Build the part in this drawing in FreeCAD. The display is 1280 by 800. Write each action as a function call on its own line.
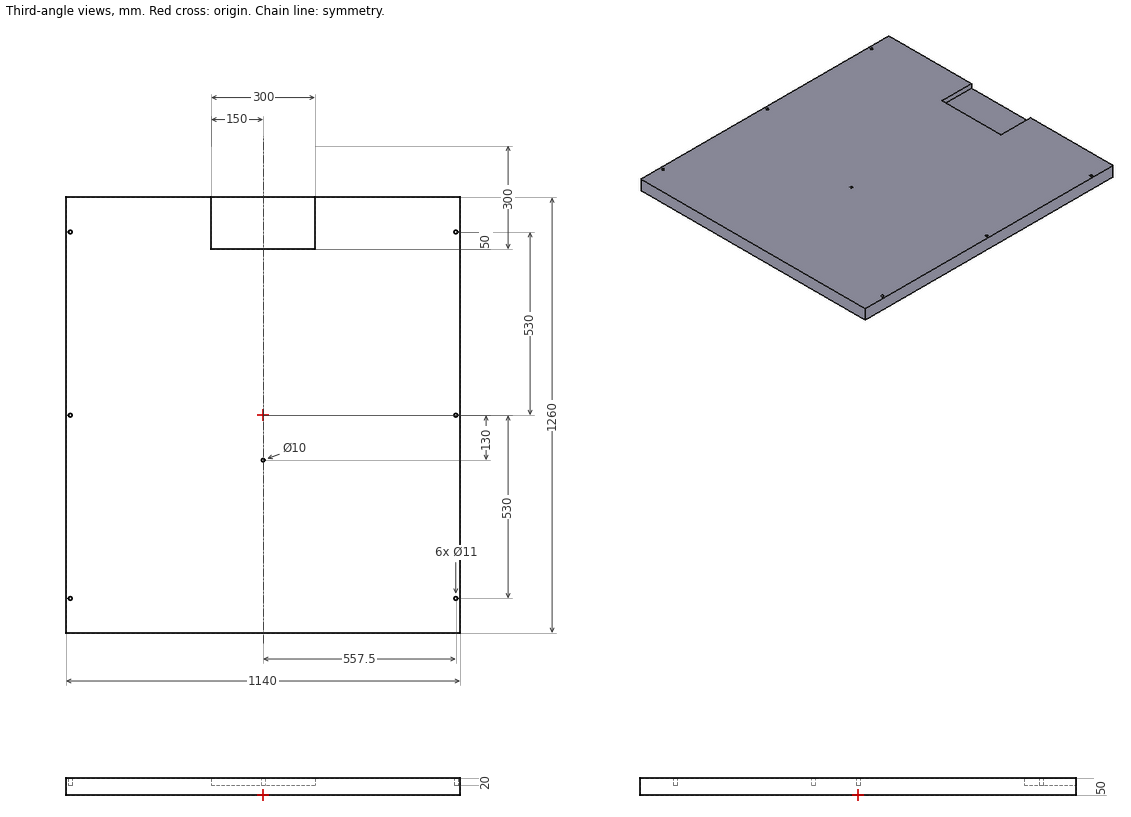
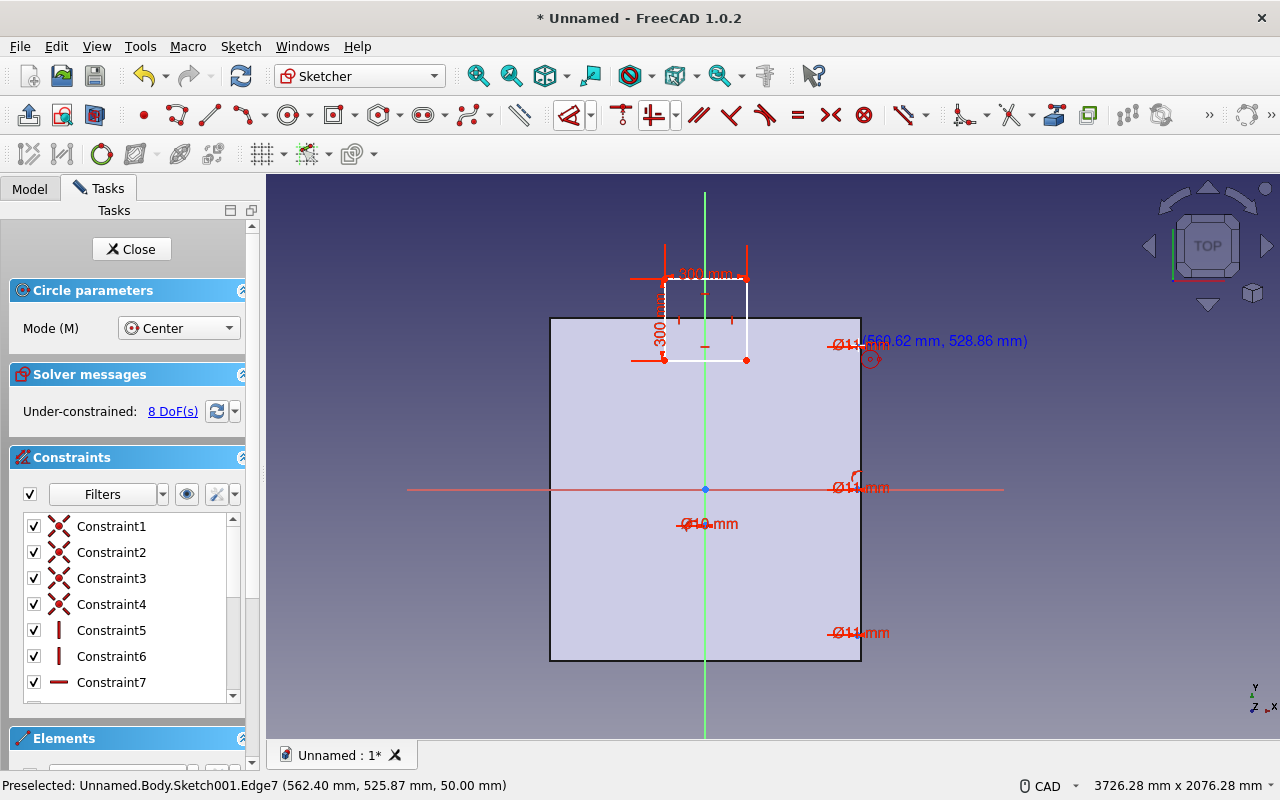
scroll(554, 346, up, 14)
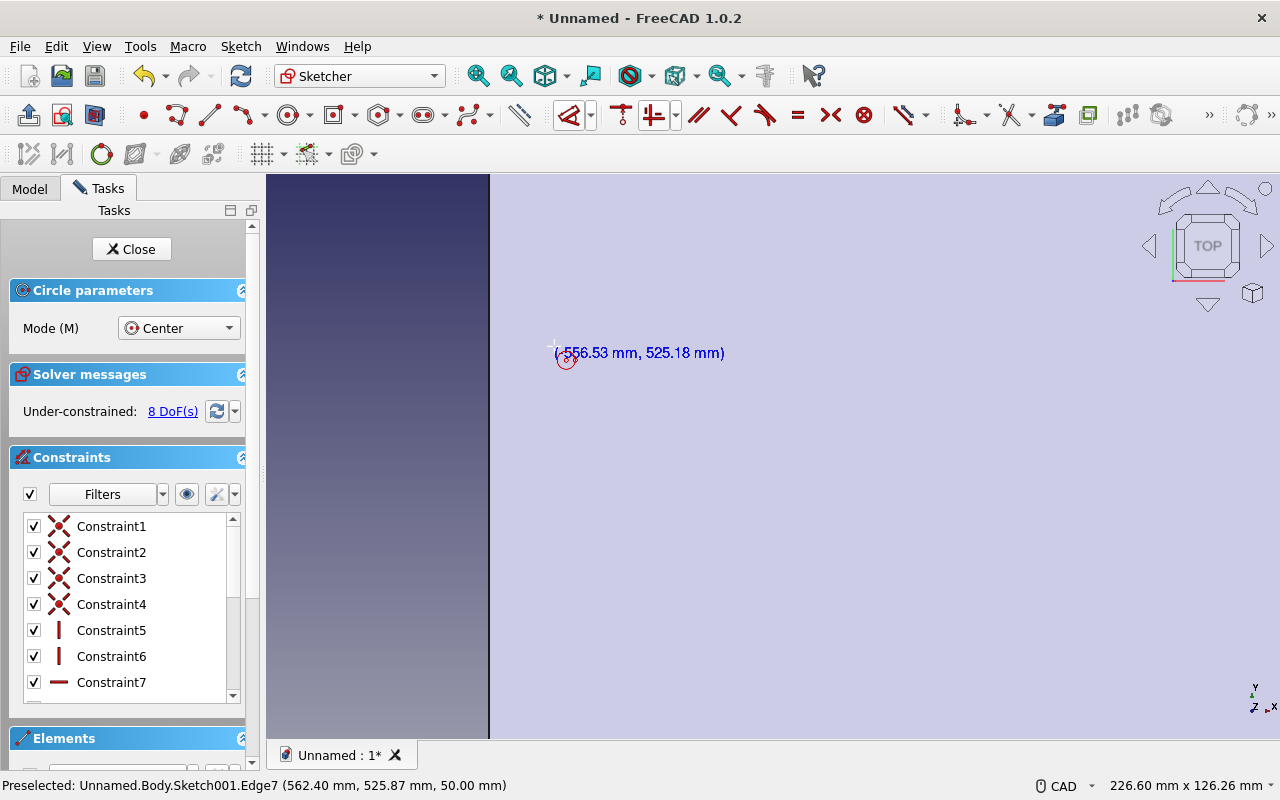
scroll(553, 346, down, 14)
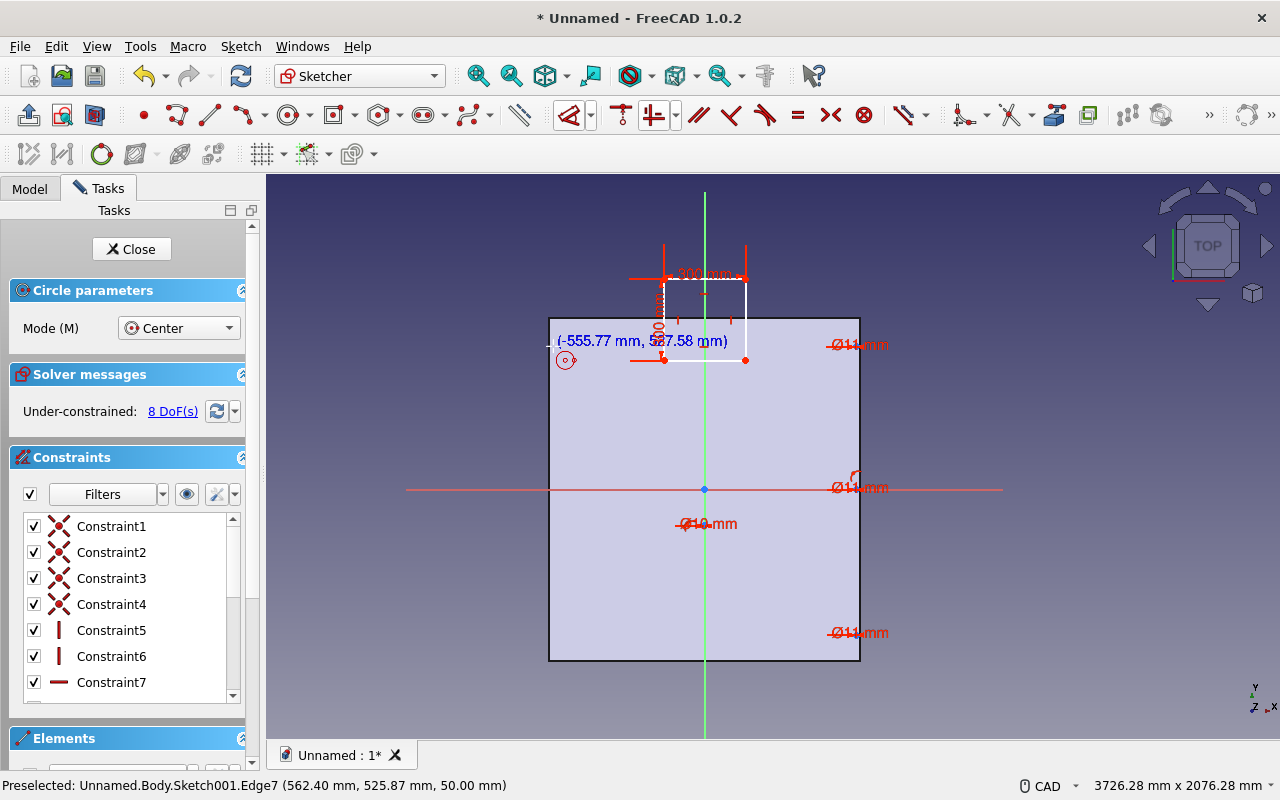
click(553, 346)
move(554, 345)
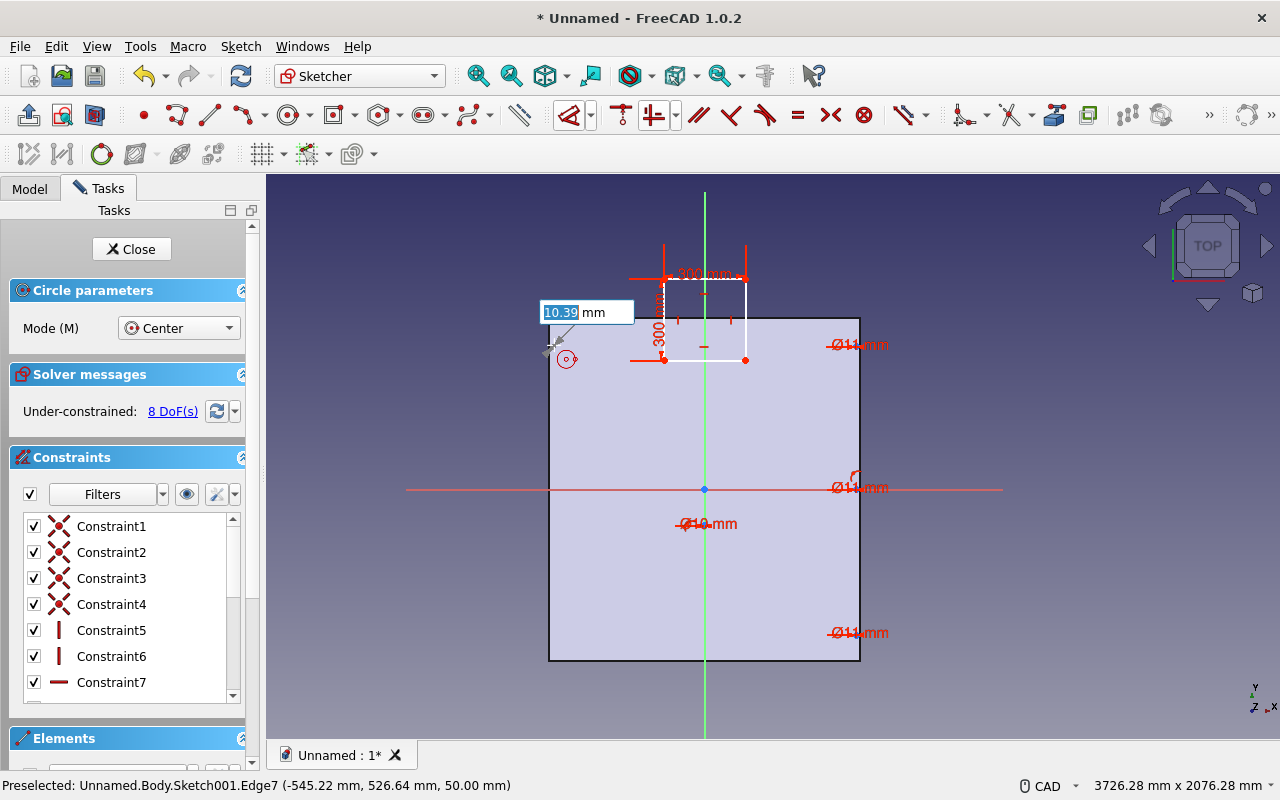
text(11)
key(Return)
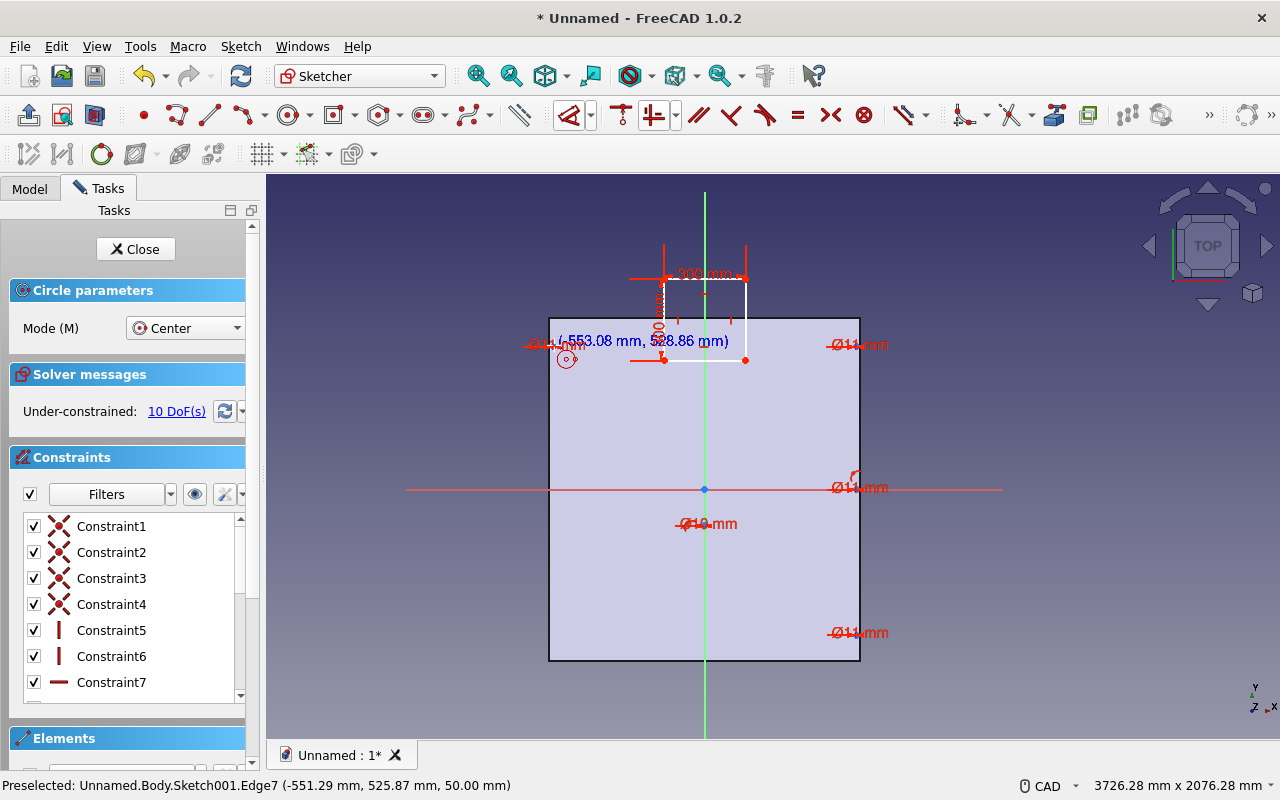
scroll(553, 490, up, 14)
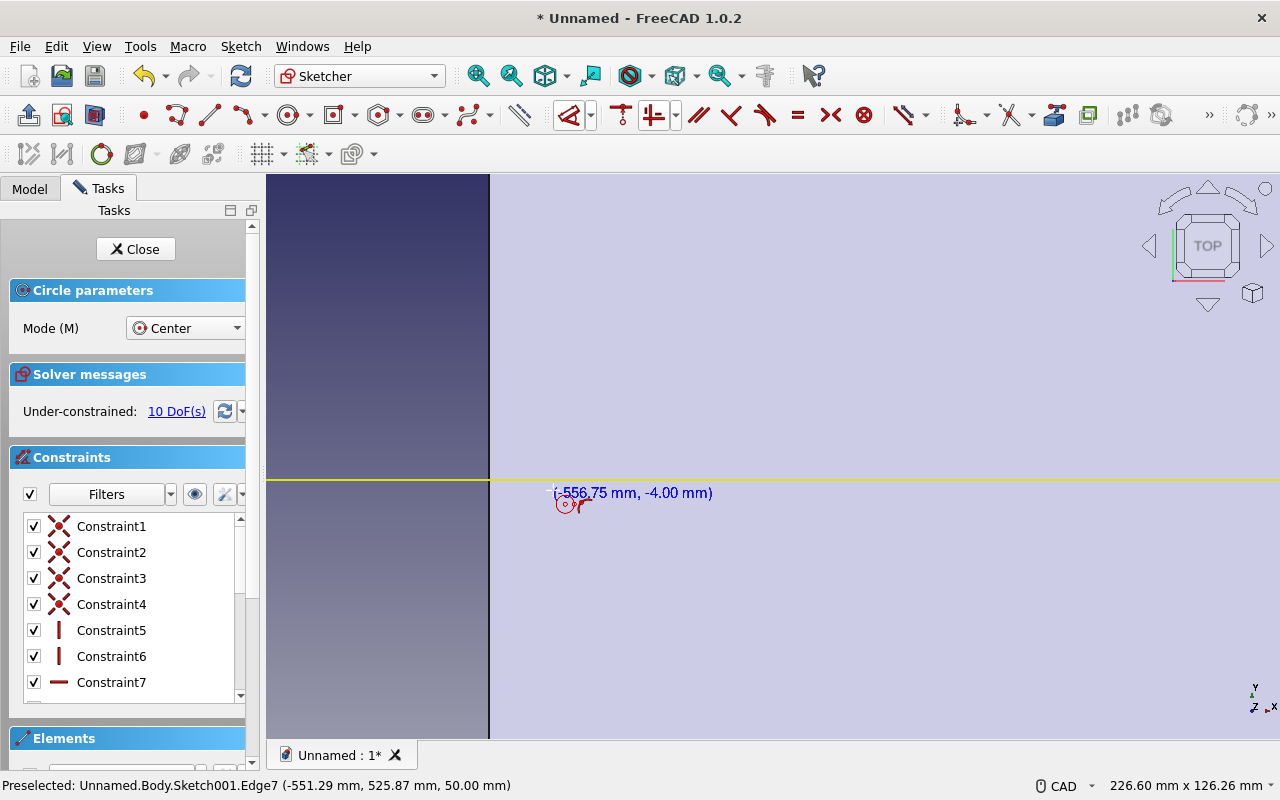
scroll(553, 490, down, 14)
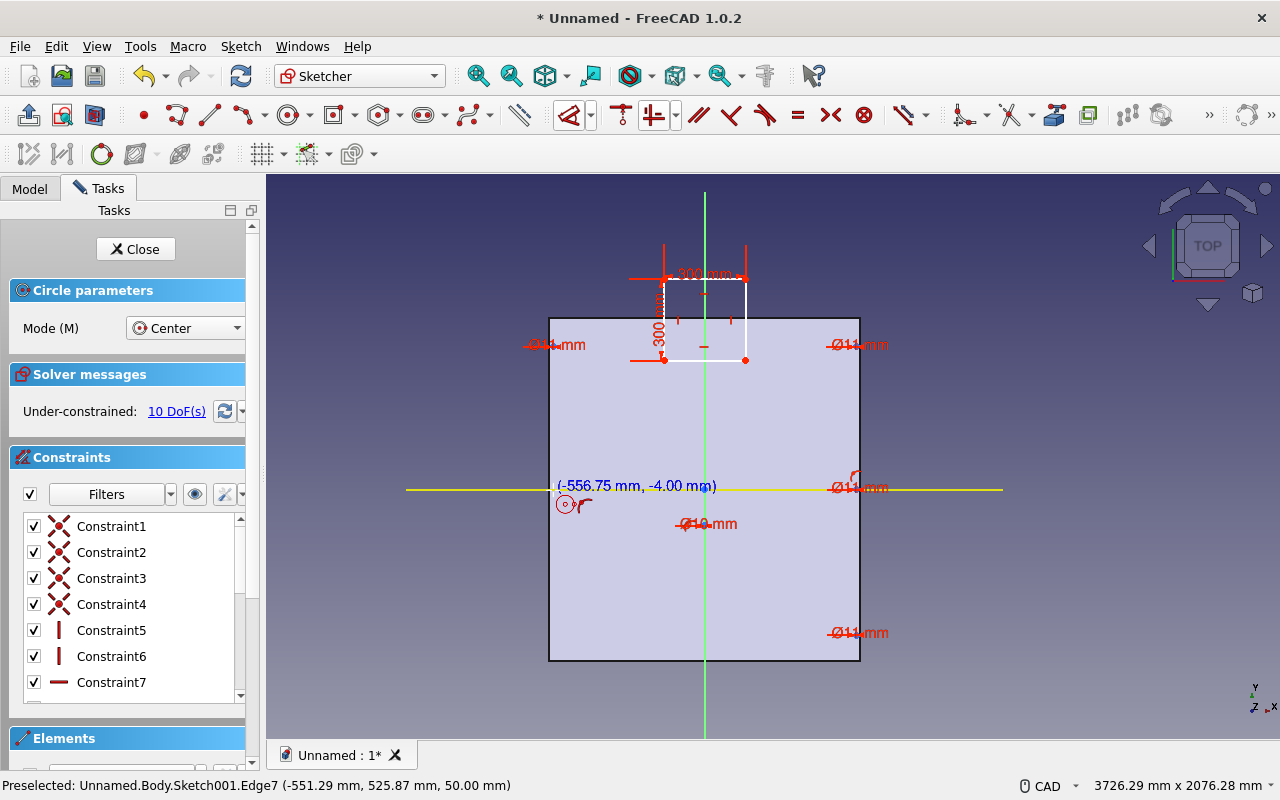
click(553, 490)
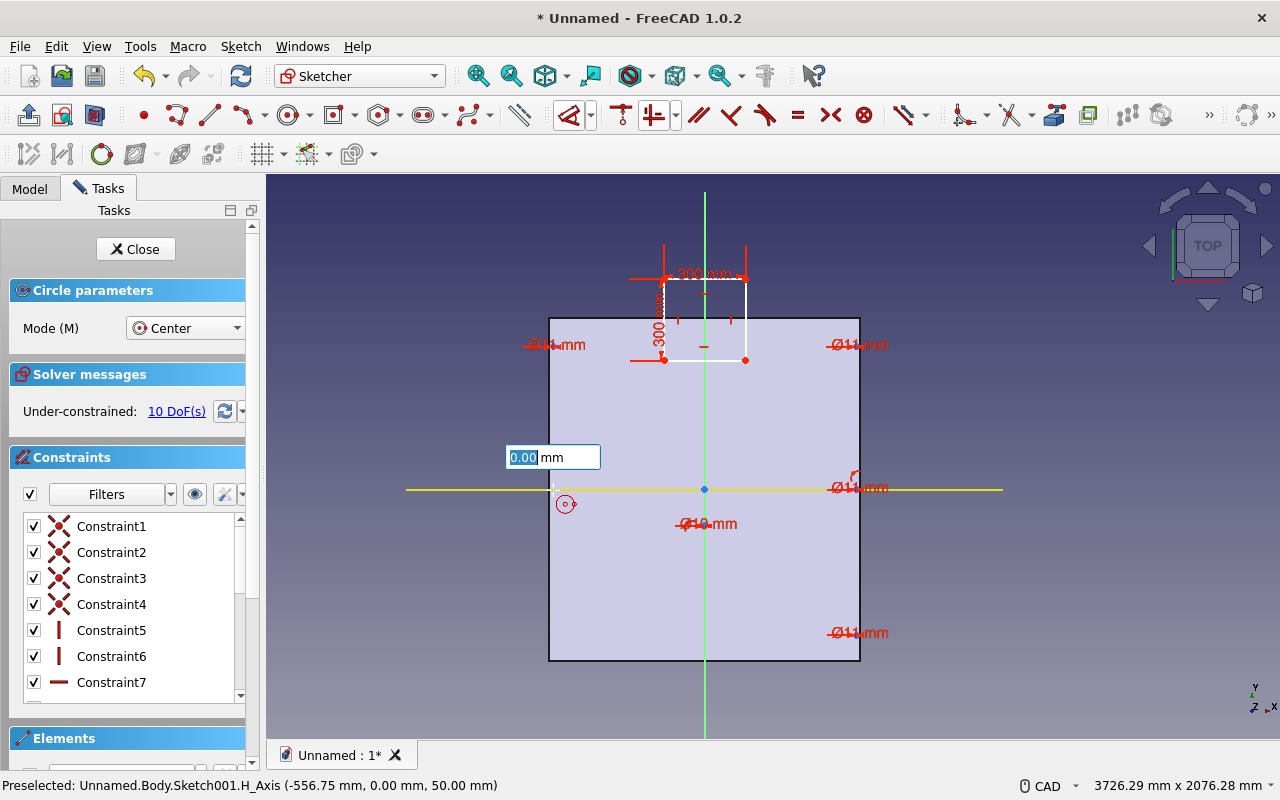
scroll(553, 489, up, 13)
move(554, 475)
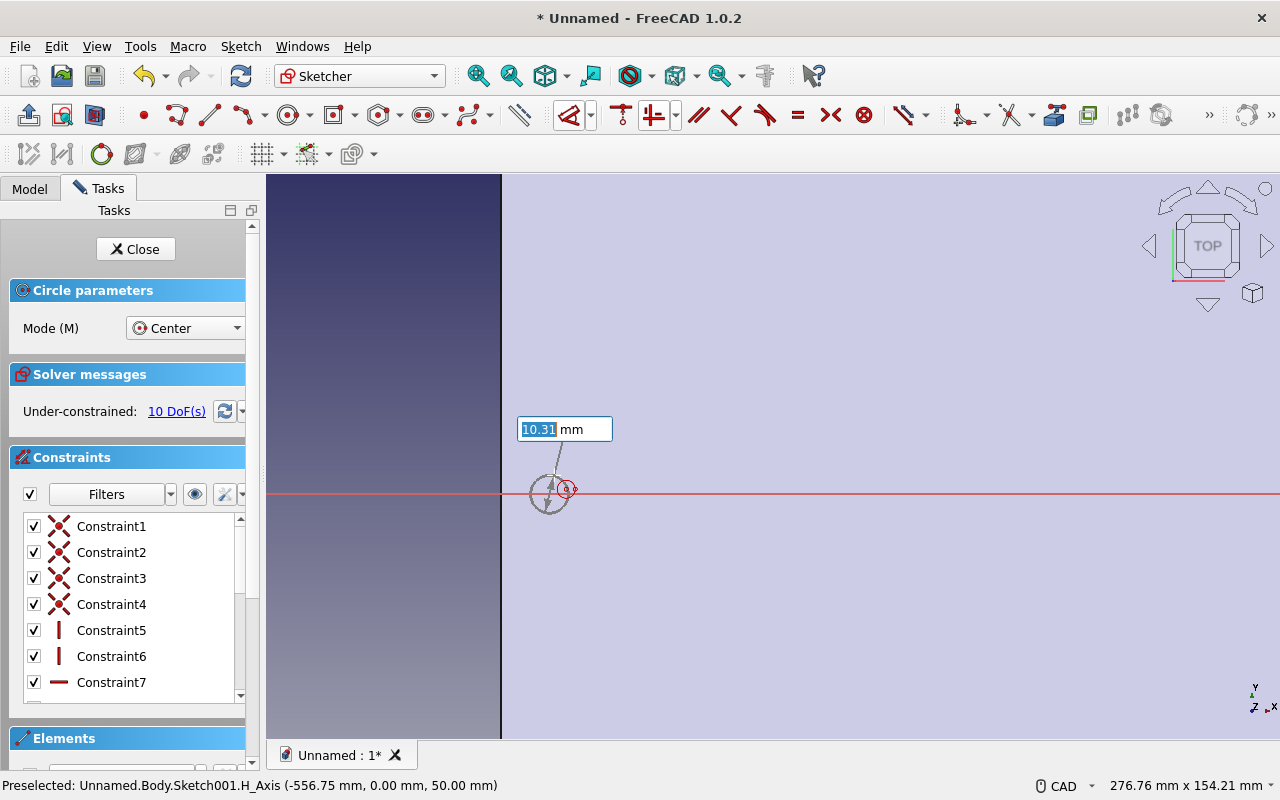
text(11)
key(Return)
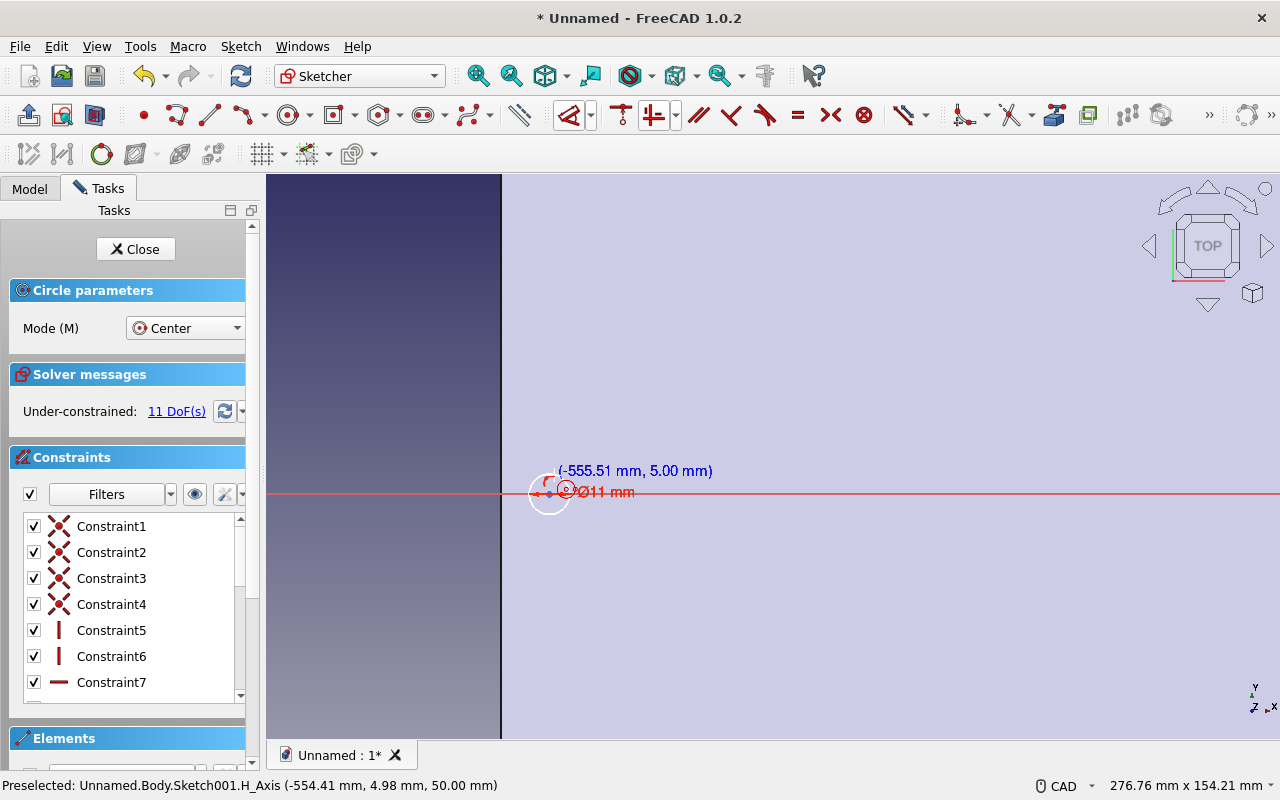
scroll(553, 489, down, 13)